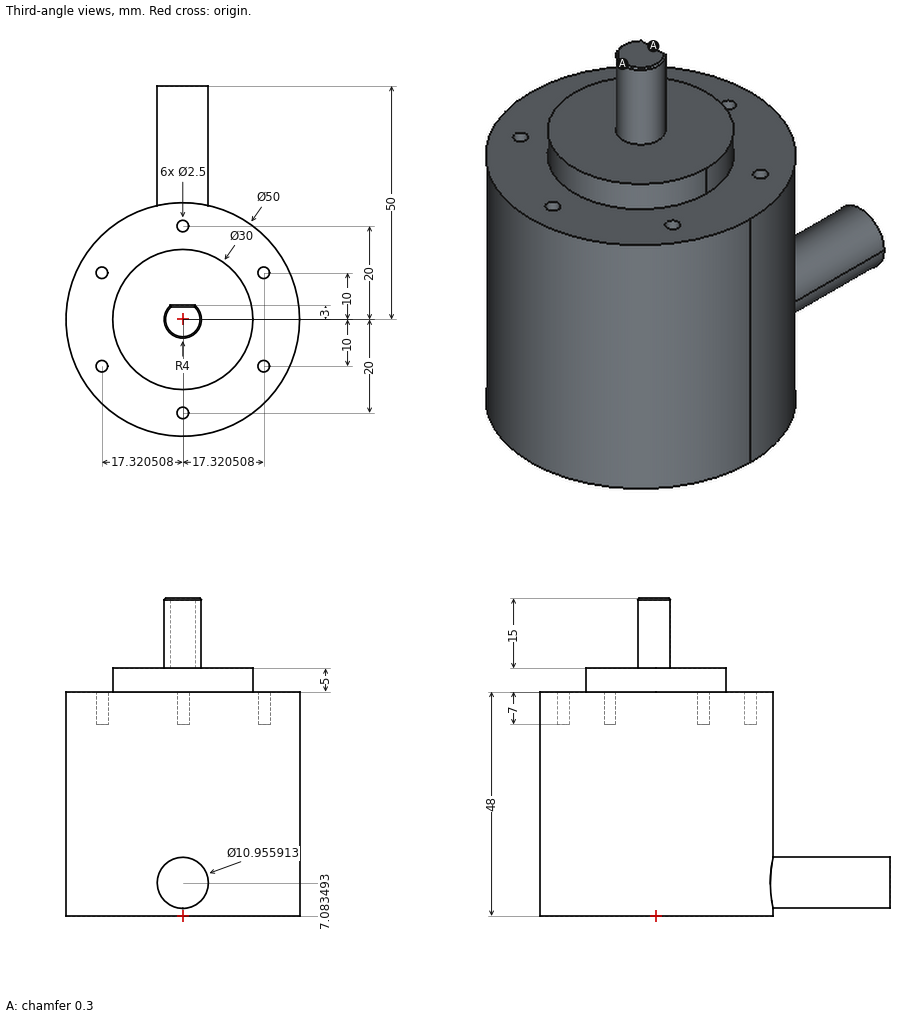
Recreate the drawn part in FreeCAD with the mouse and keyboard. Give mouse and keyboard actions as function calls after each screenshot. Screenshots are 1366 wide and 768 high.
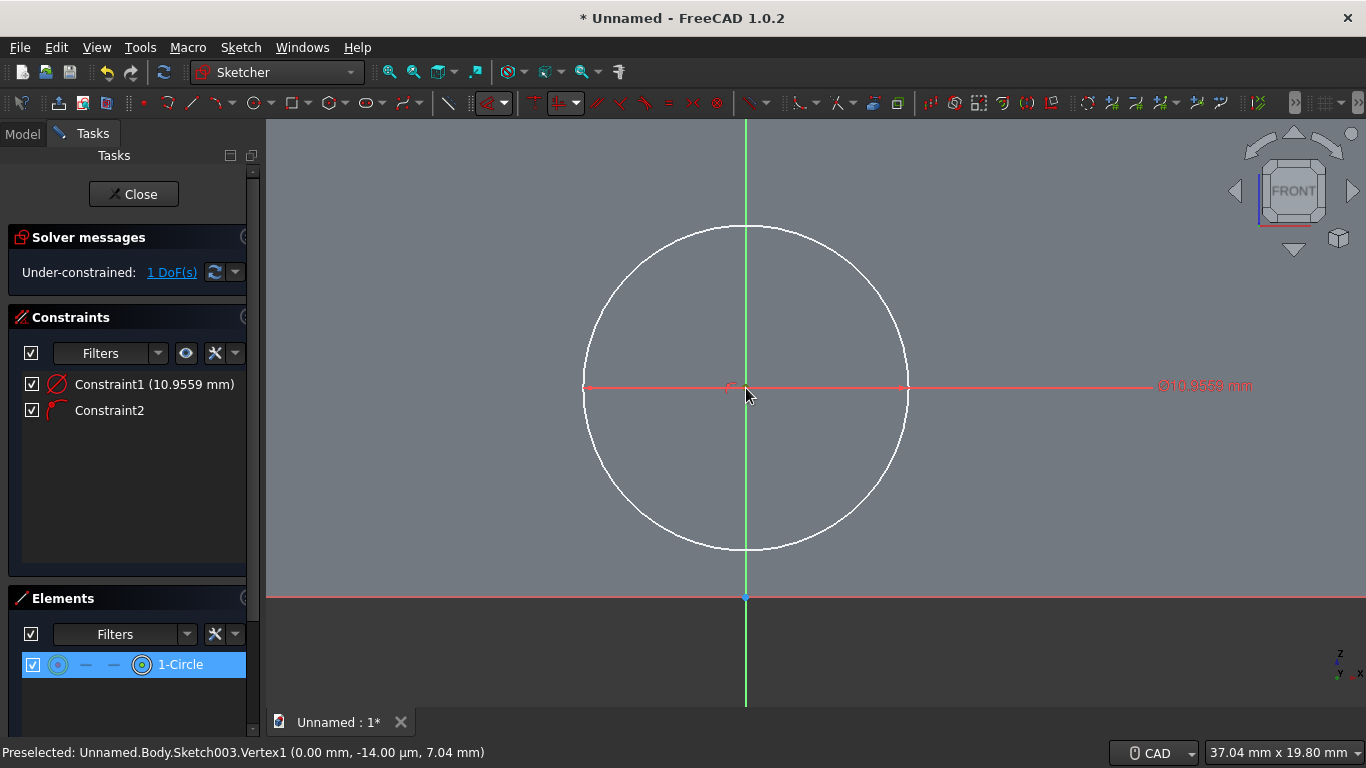
click(506, 104)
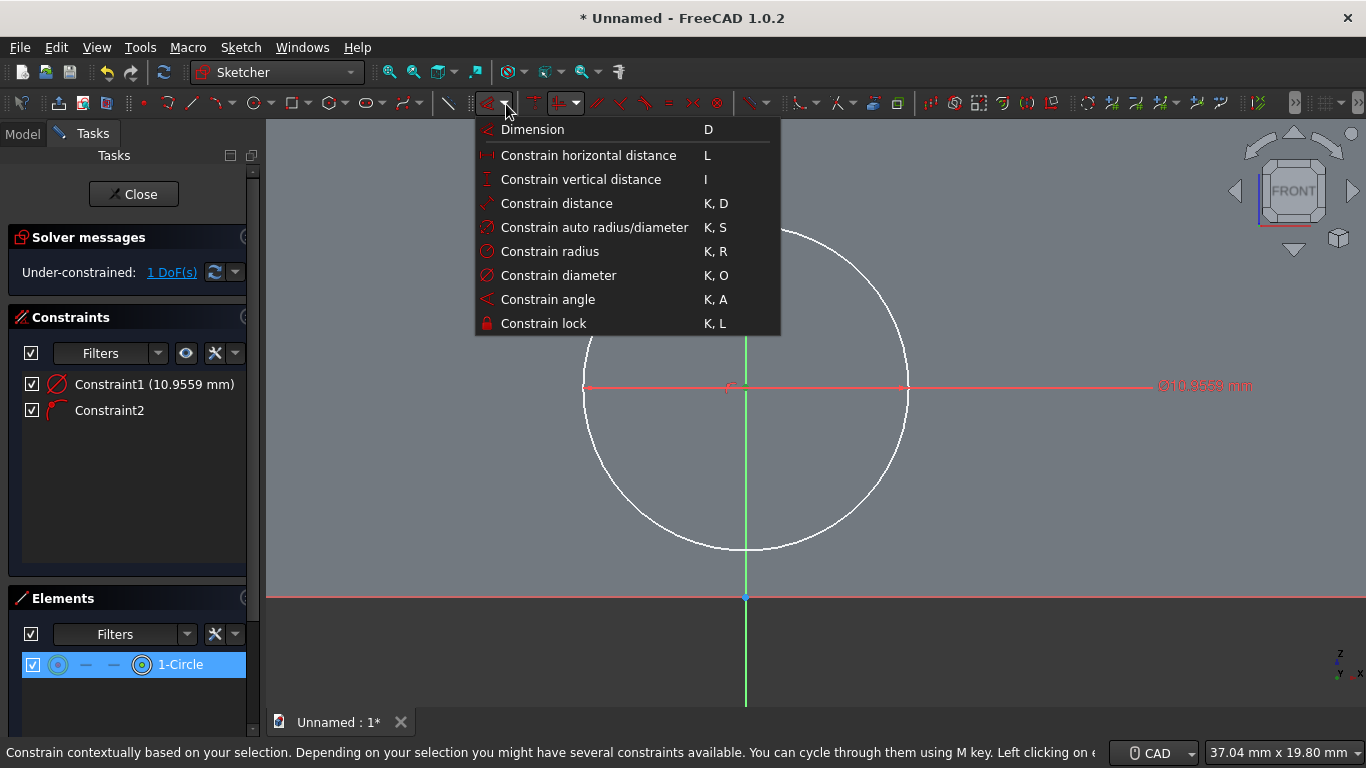
click(628, 179)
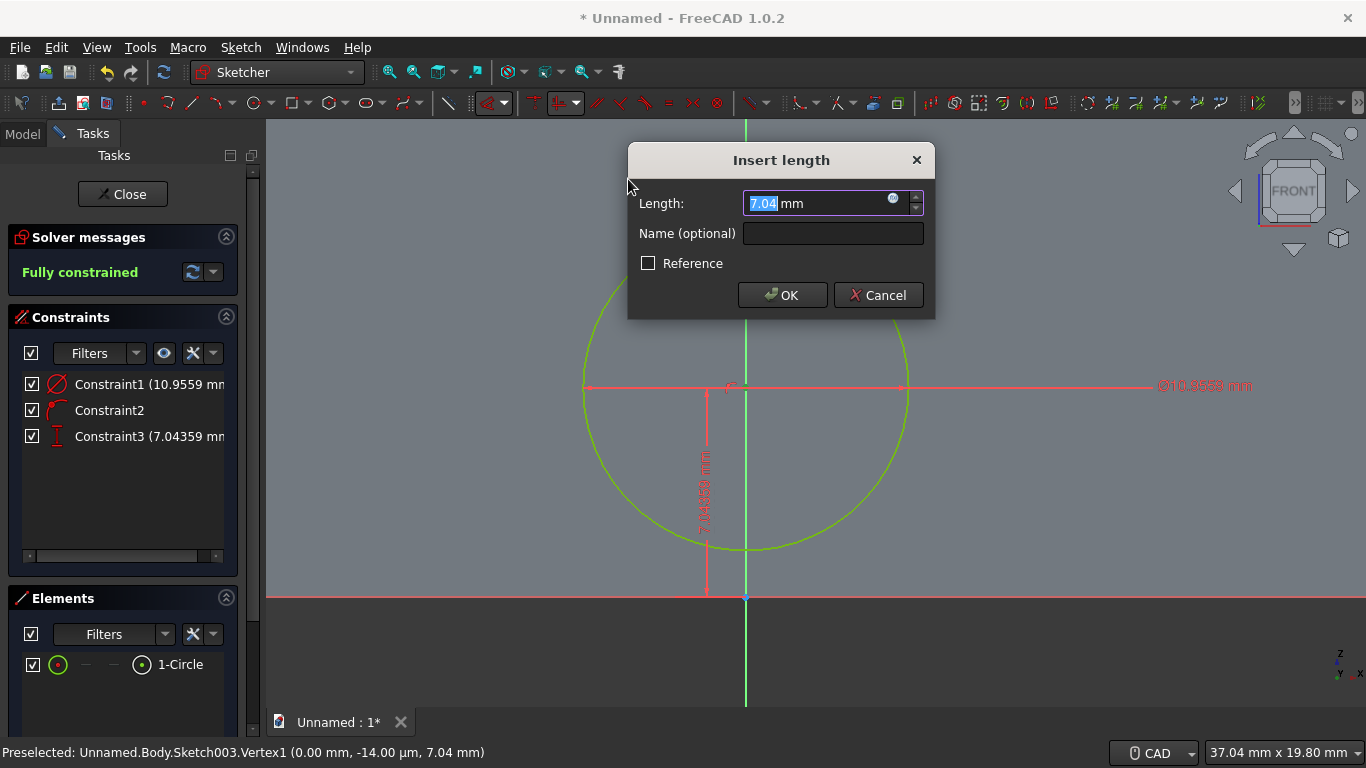
text(7.083493)
key(Return)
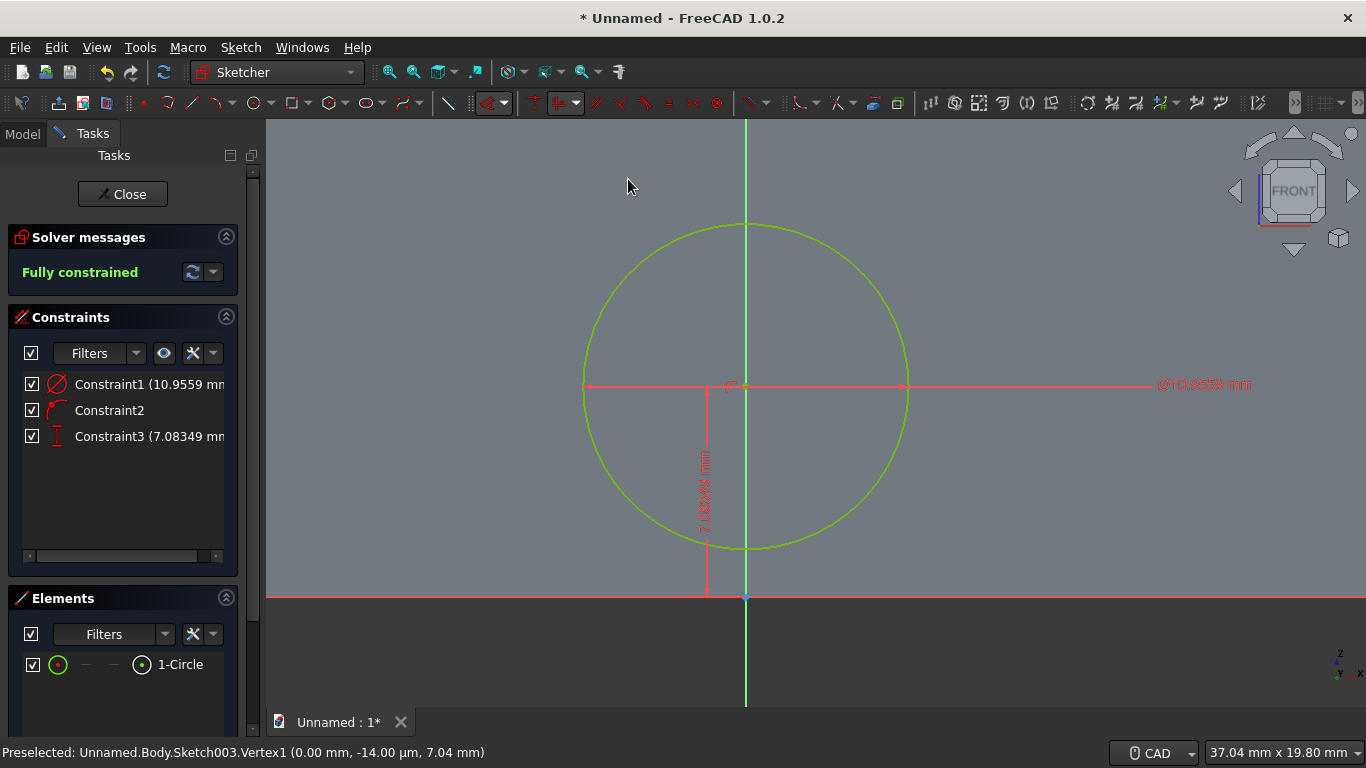
click(123, 194)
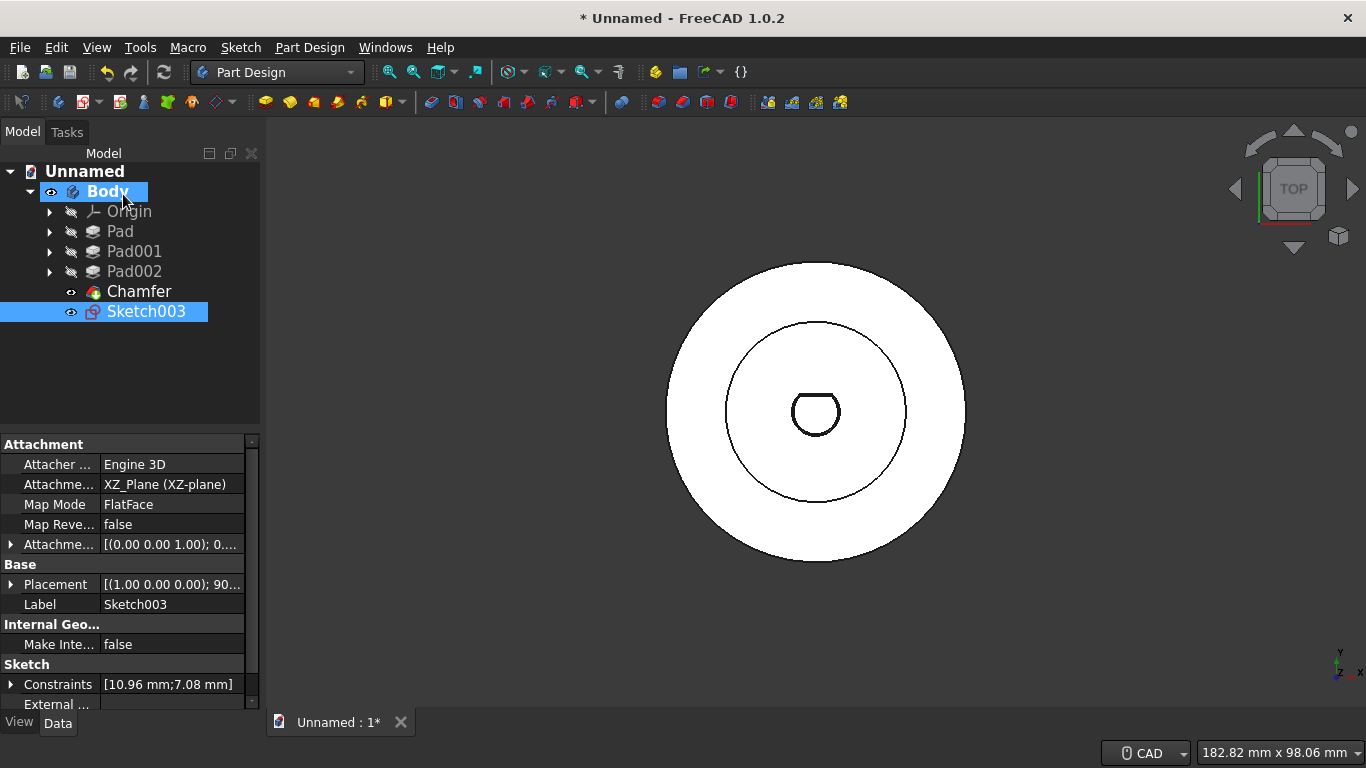
click(266, 102)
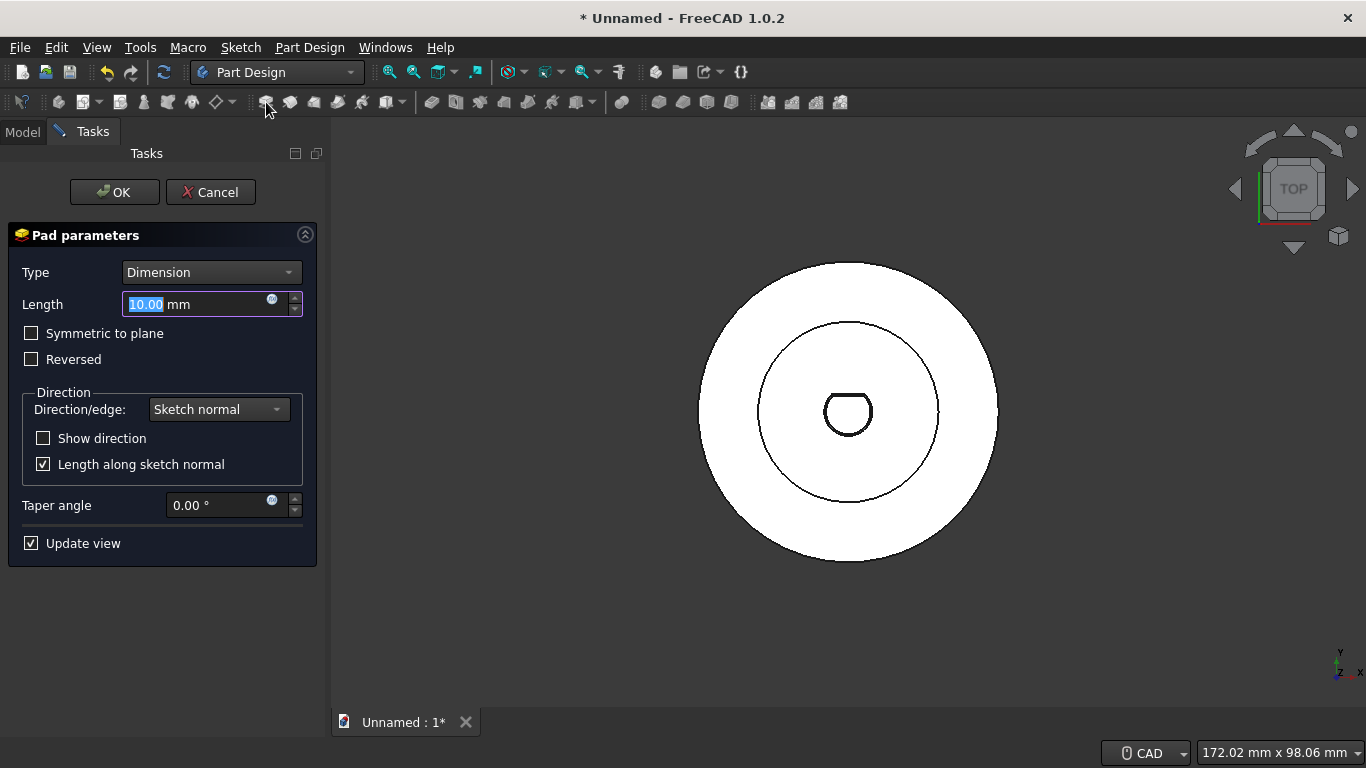
text(50)
key(Tab)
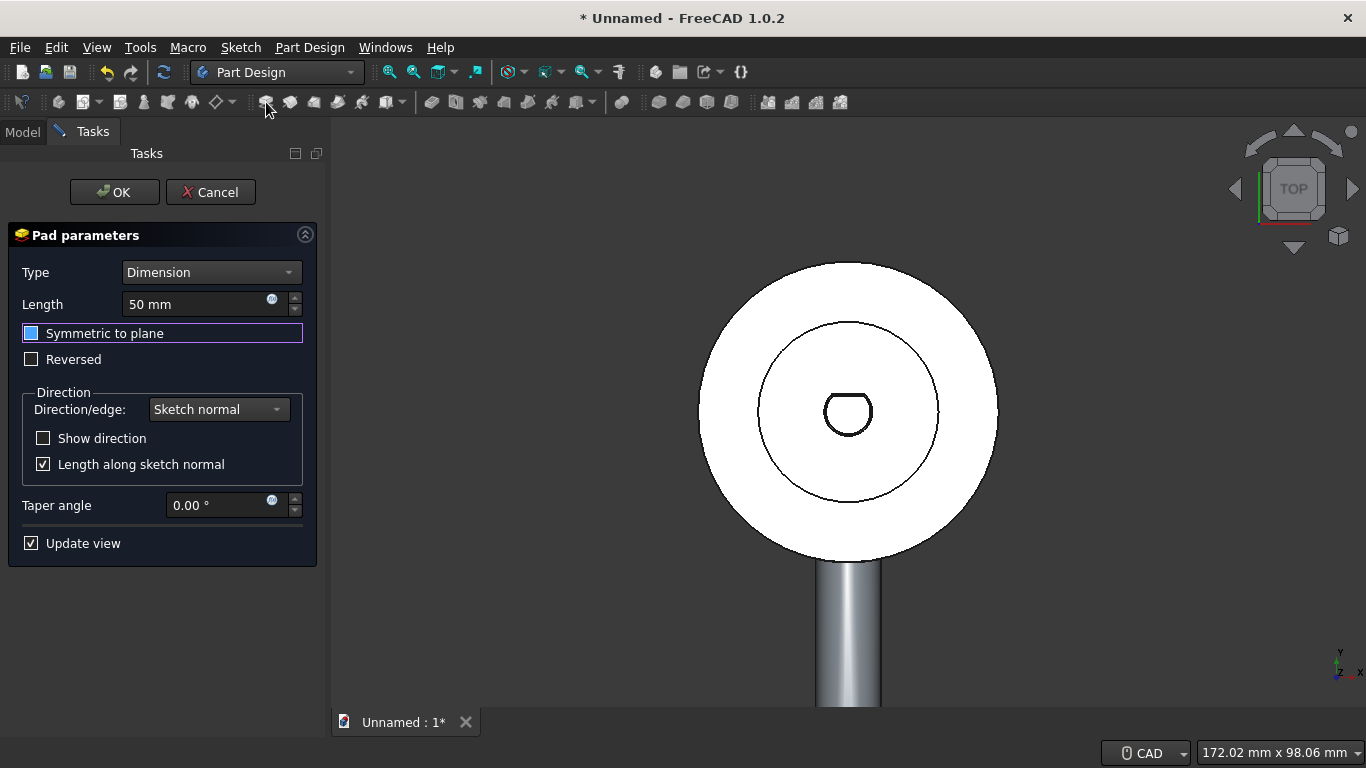
click(30, 359)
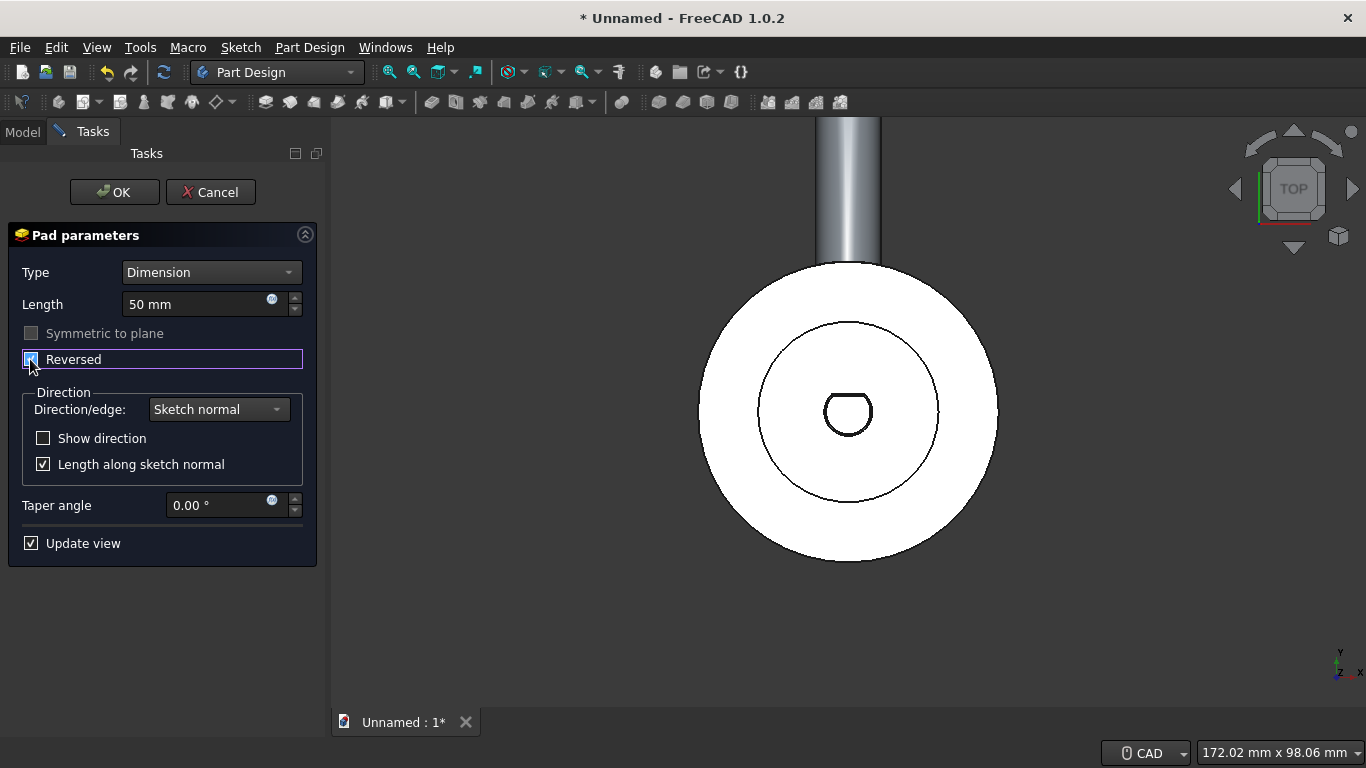
click(115, 192)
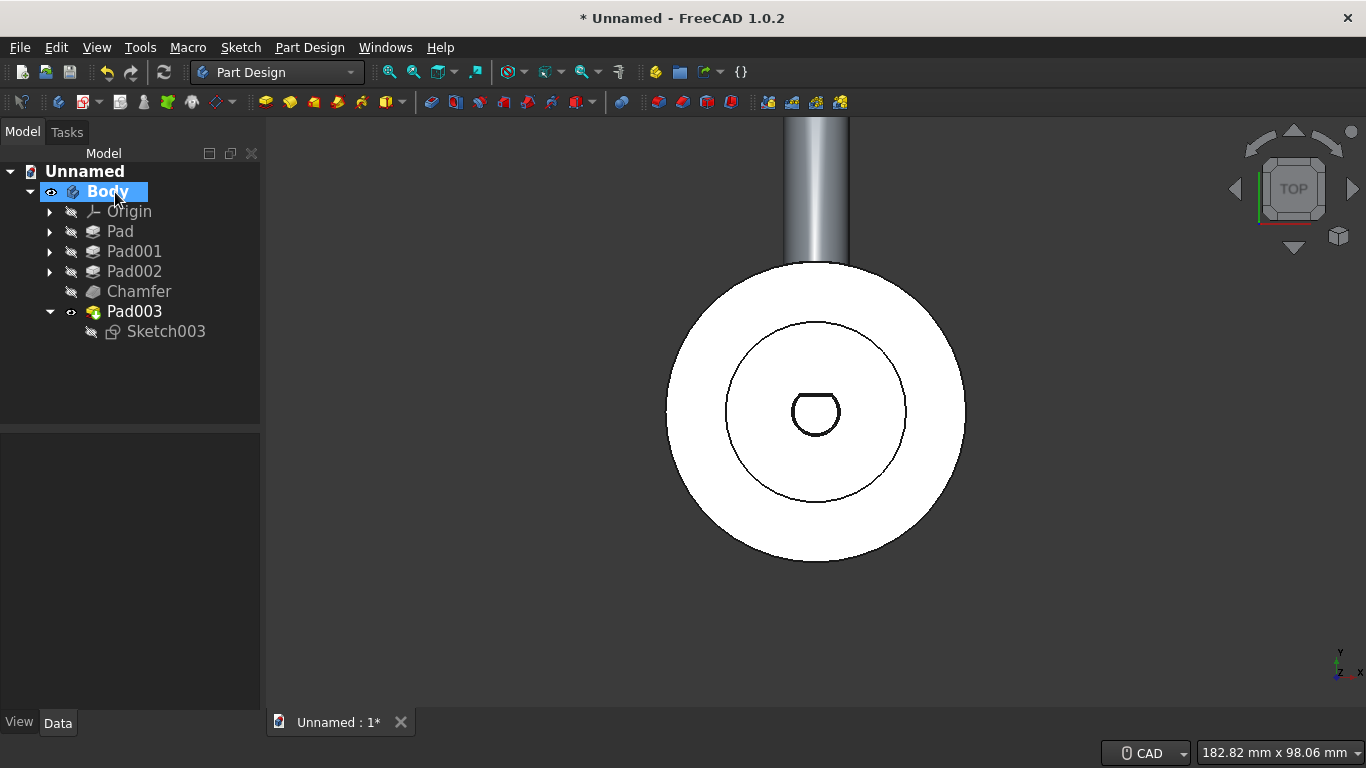
click(390, 72)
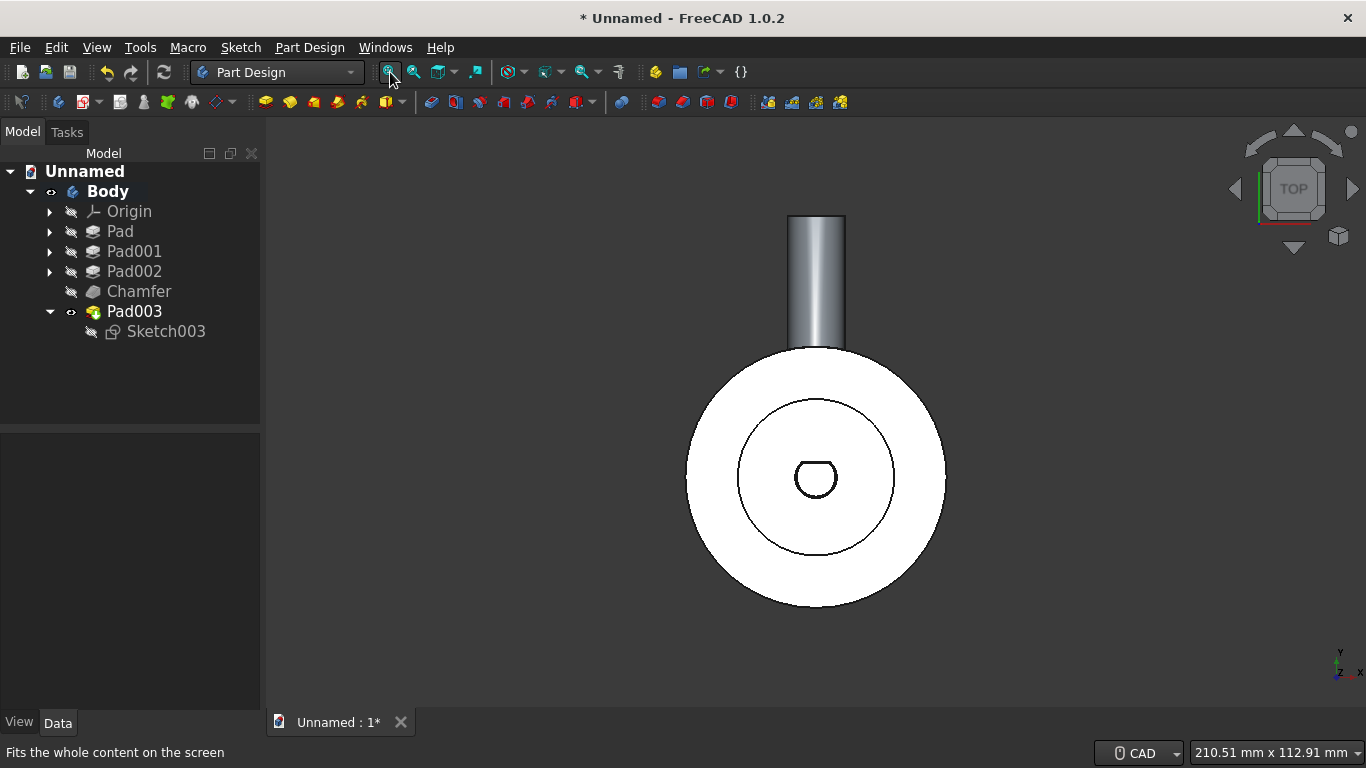
click(891, 551)